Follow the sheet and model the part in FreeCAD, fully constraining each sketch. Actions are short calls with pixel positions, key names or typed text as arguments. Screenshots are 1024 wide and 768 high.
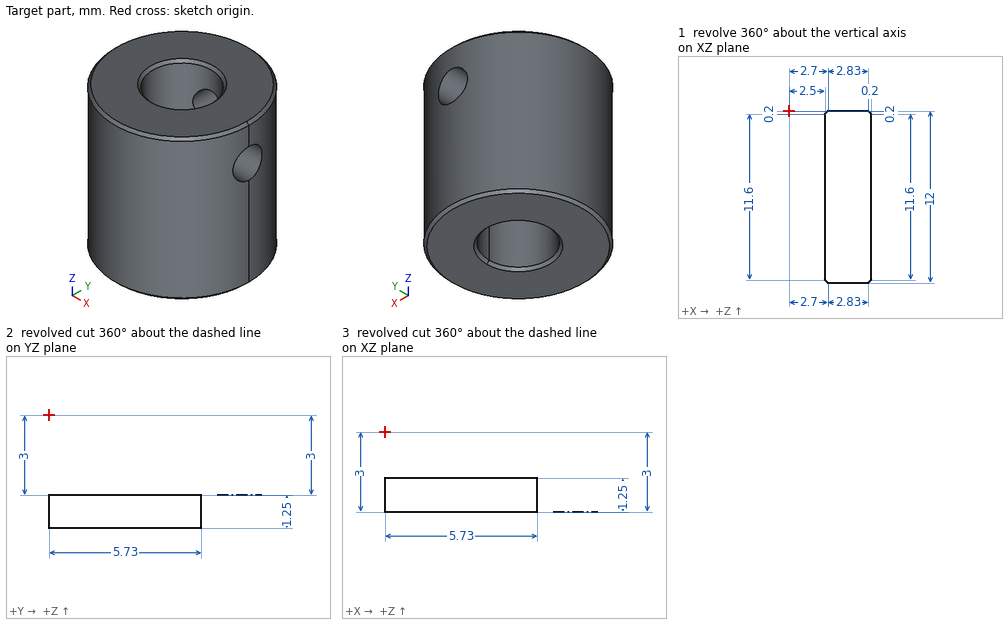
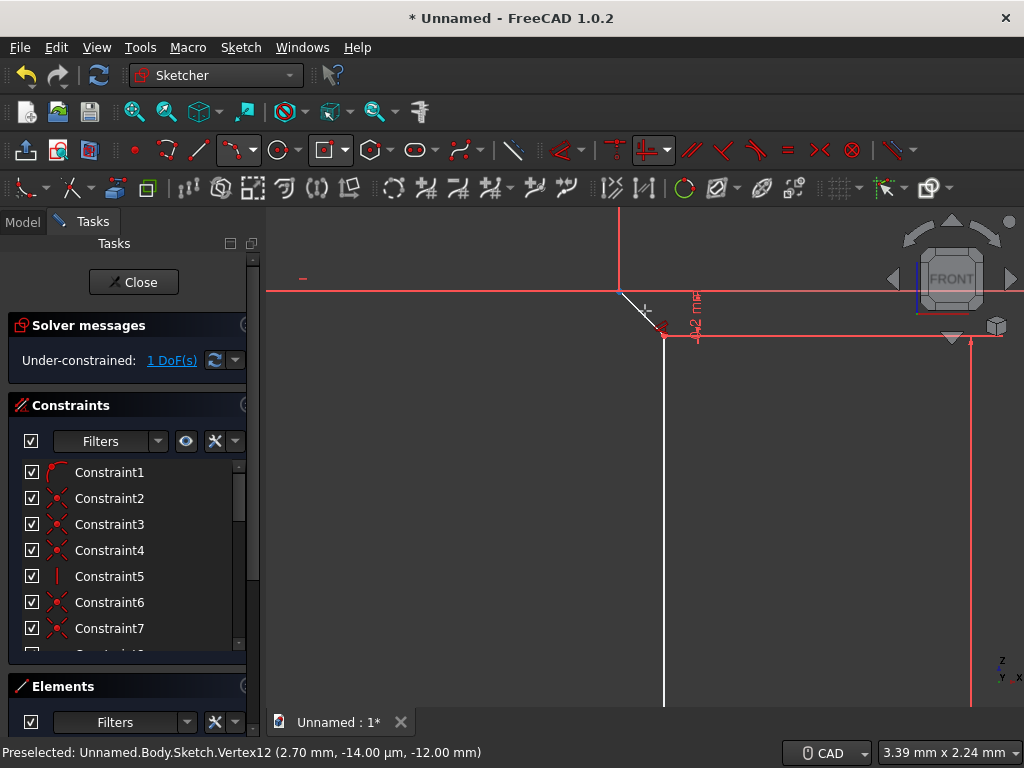
click(637, 309)
click(642, 257)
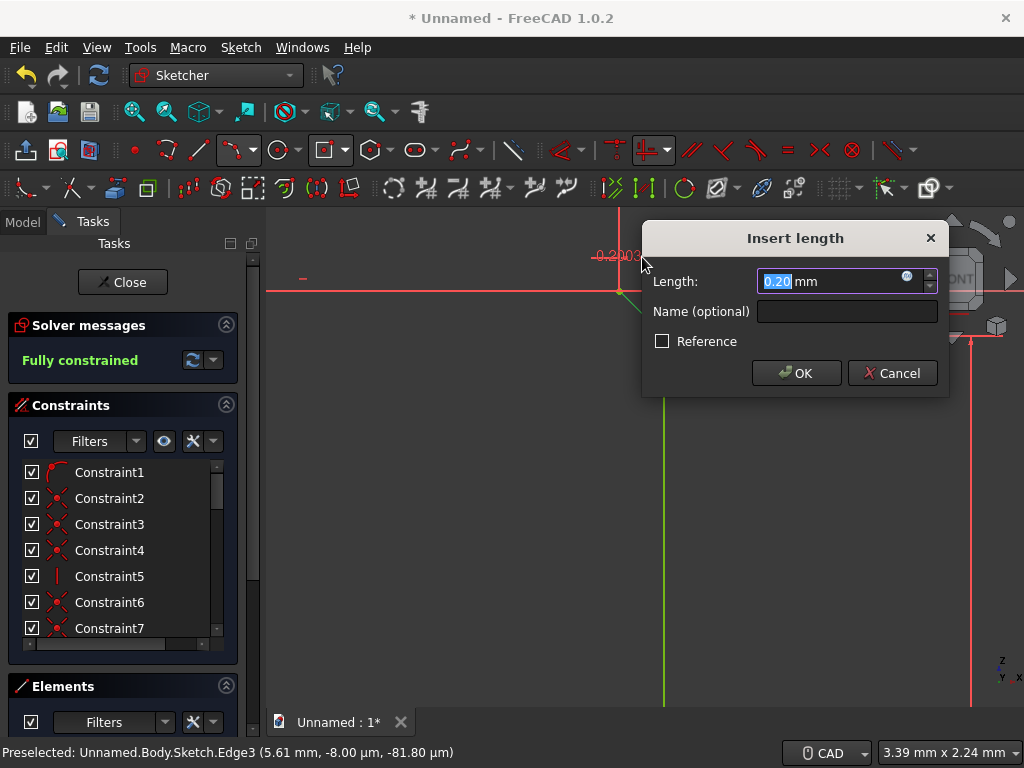
text(0.2)
key(Return)
key(Escape)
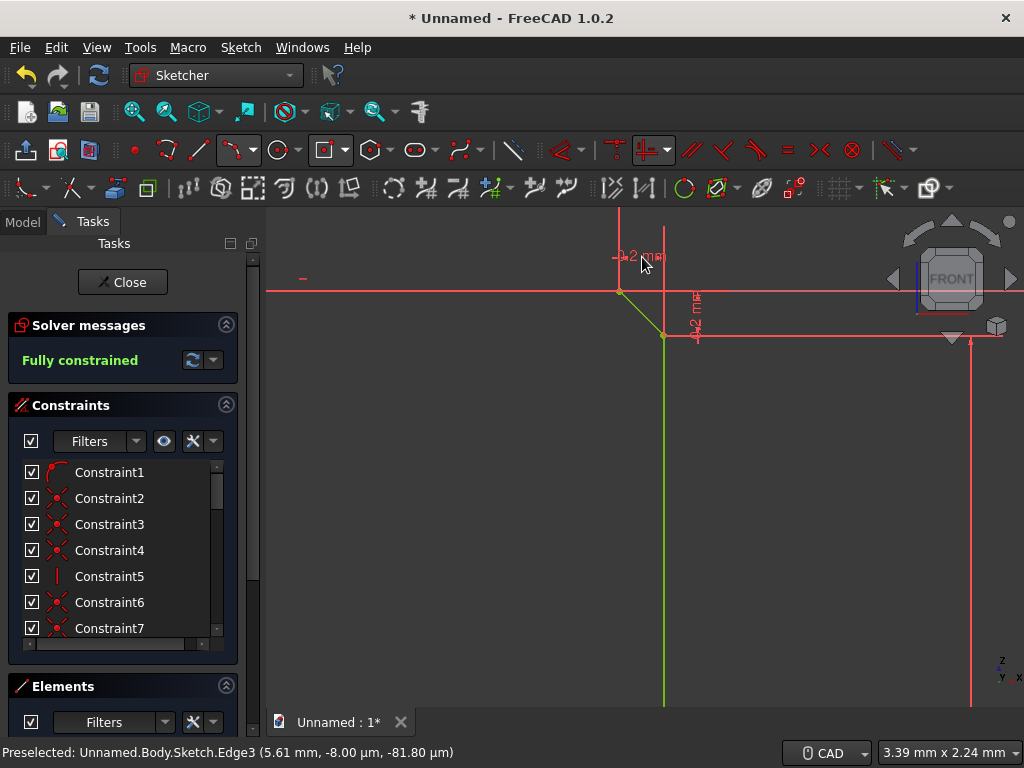
click(123, 282)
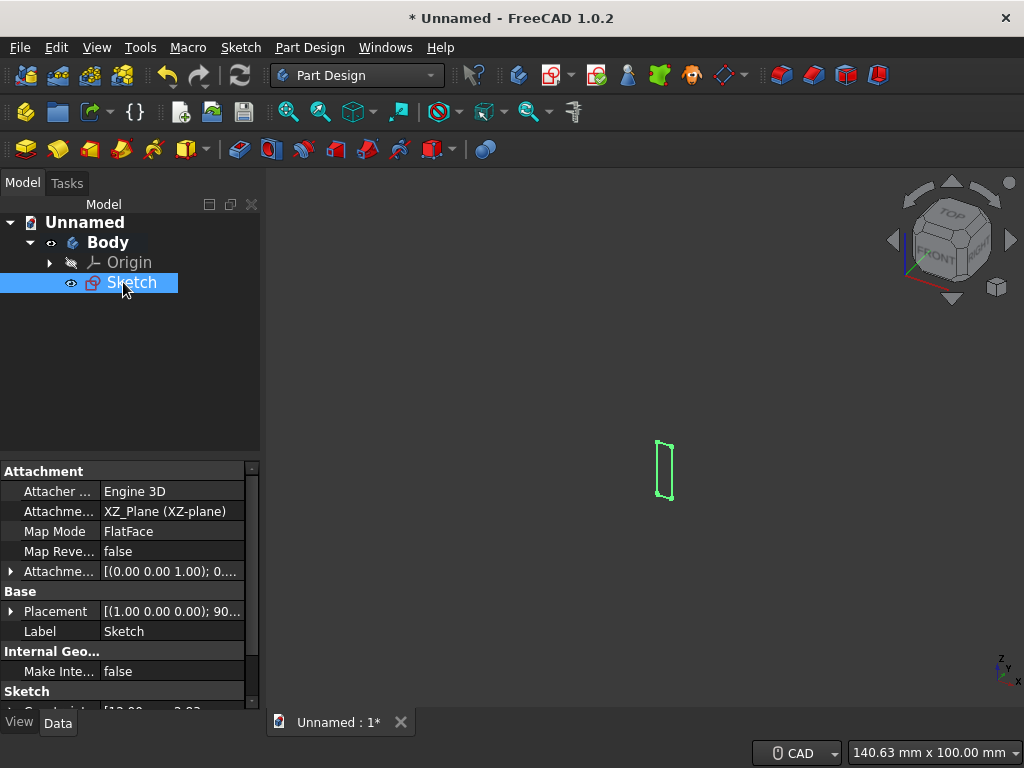
click(58, 150)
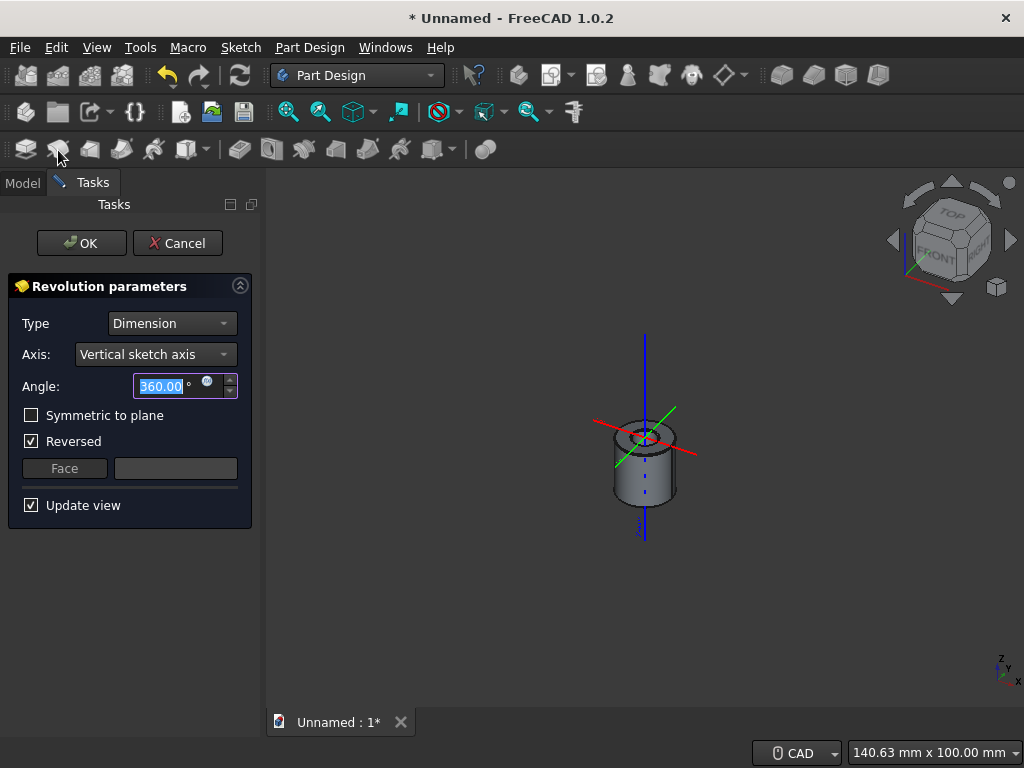
click(82, 243)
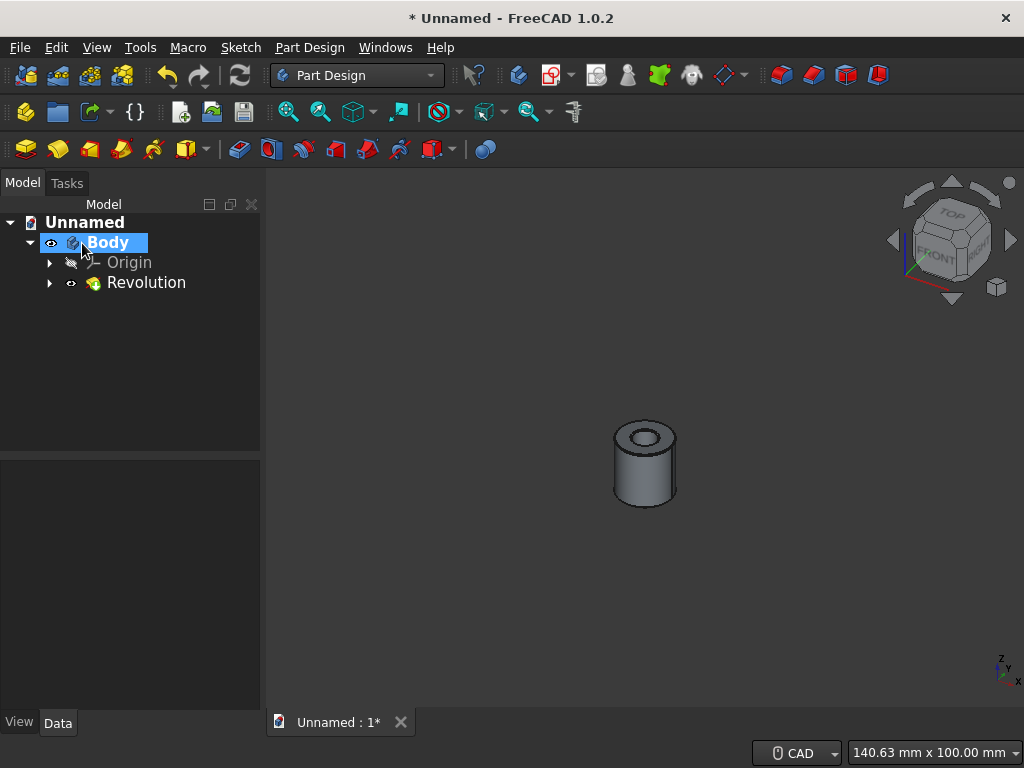
click(290, 112)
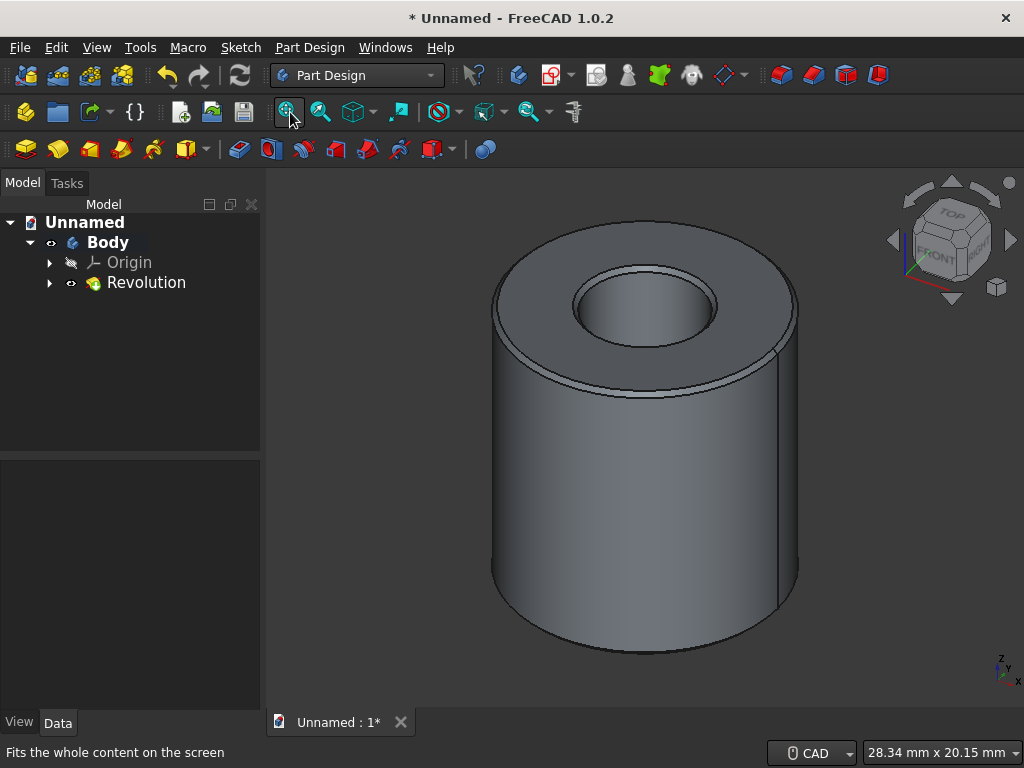
click(552, 76)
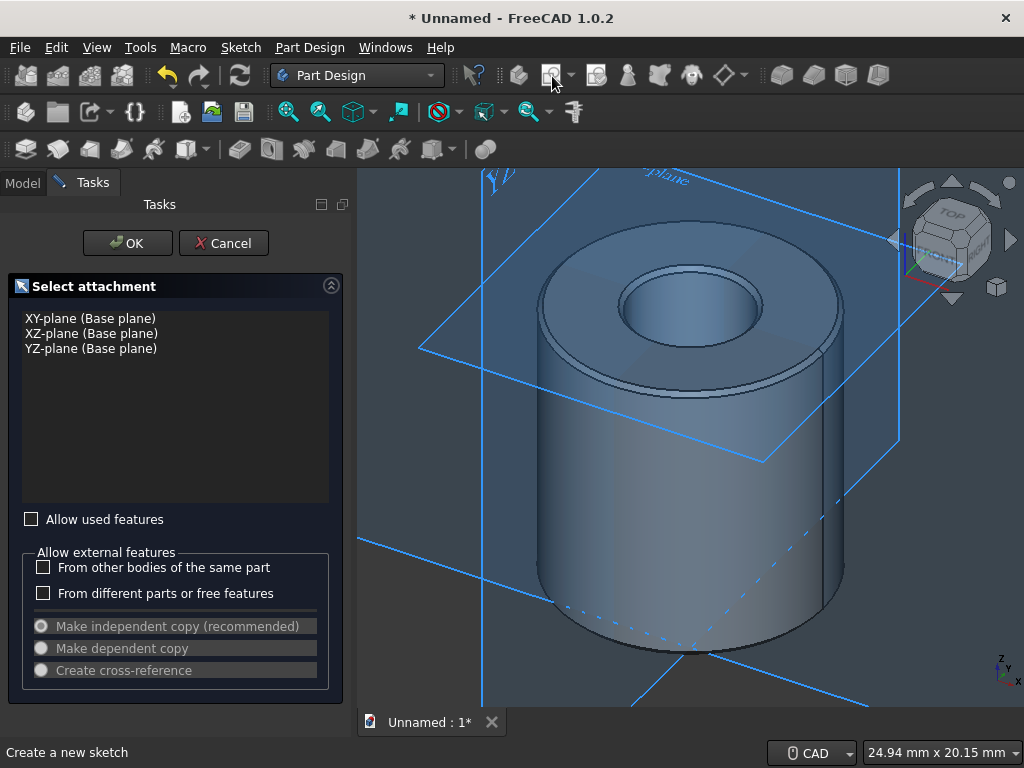
click(82, 348)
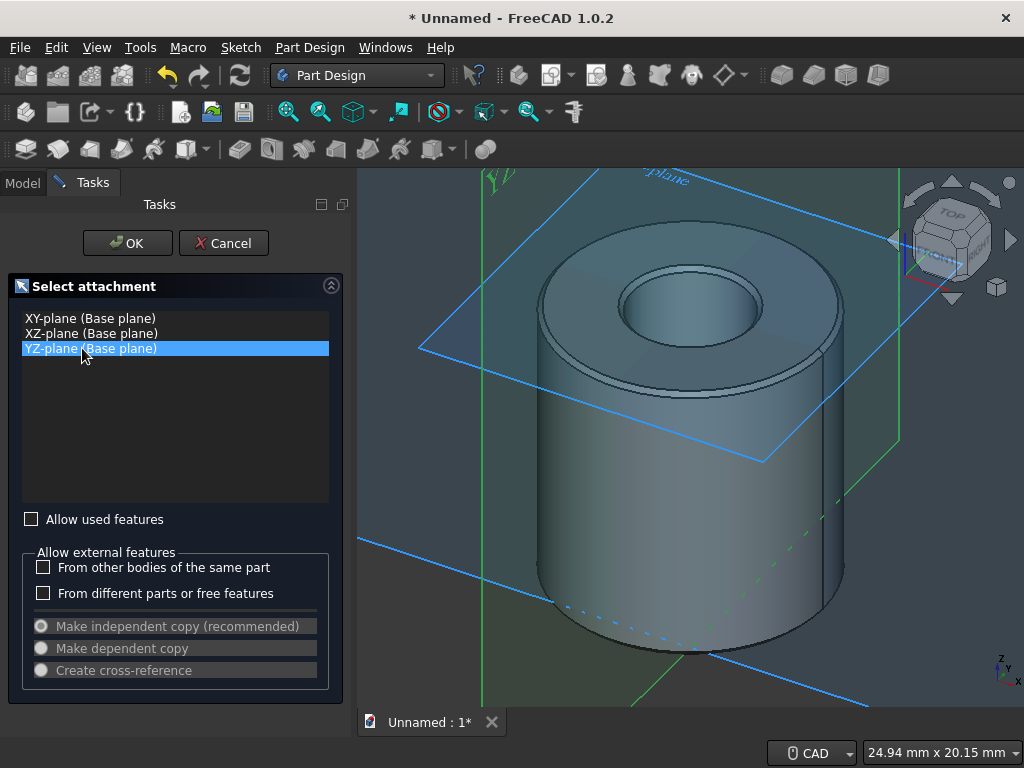
click(128, 243)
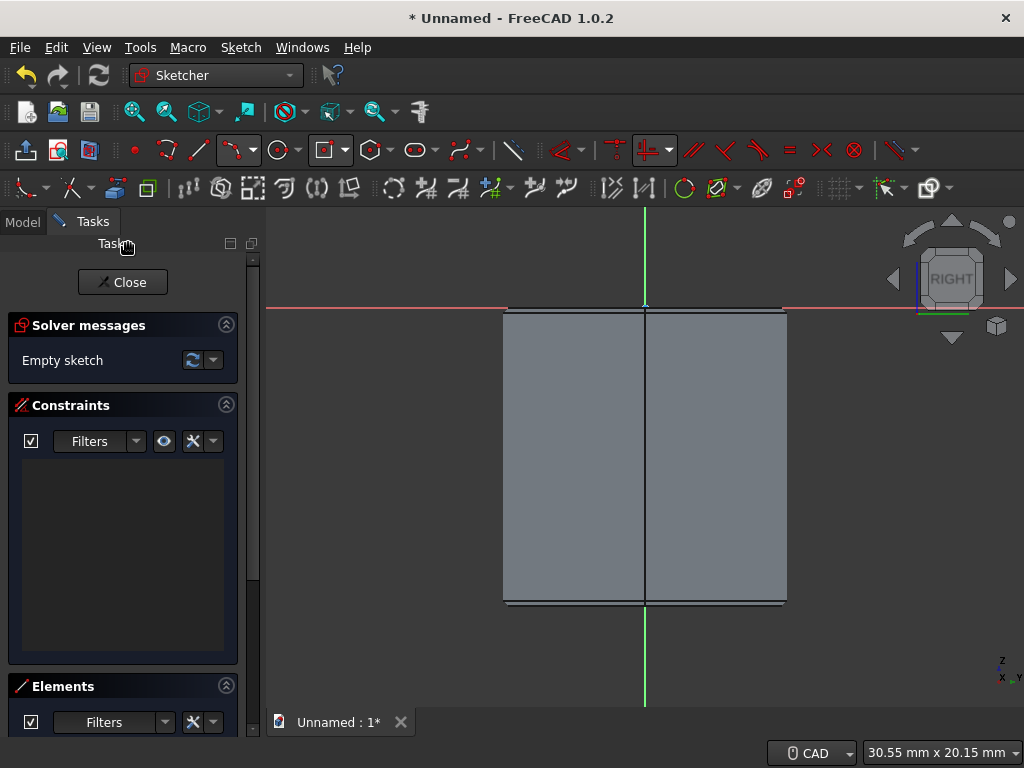
click(90, 150)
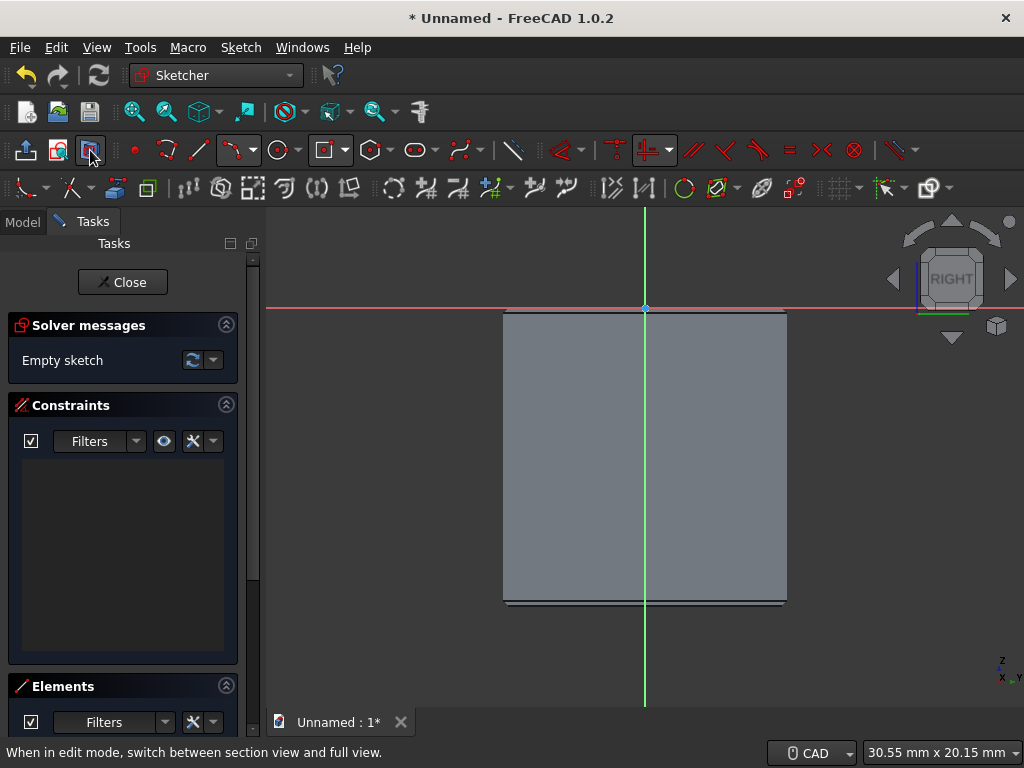
scroll(859, 244, up, 3)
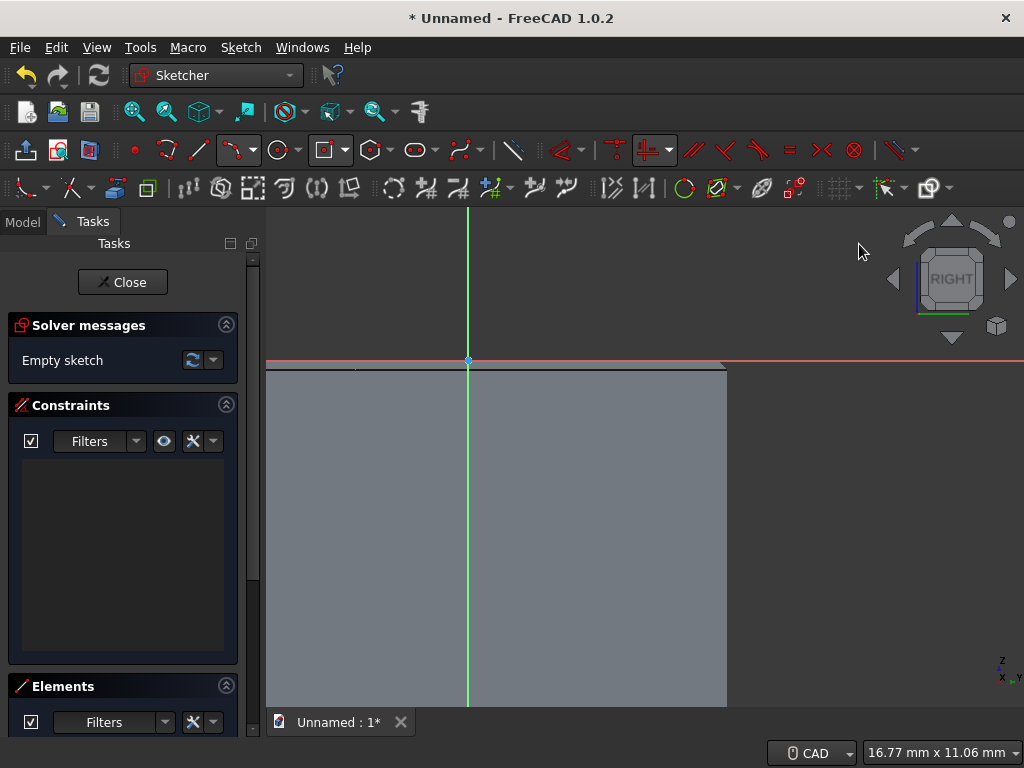
key(g)
key(r)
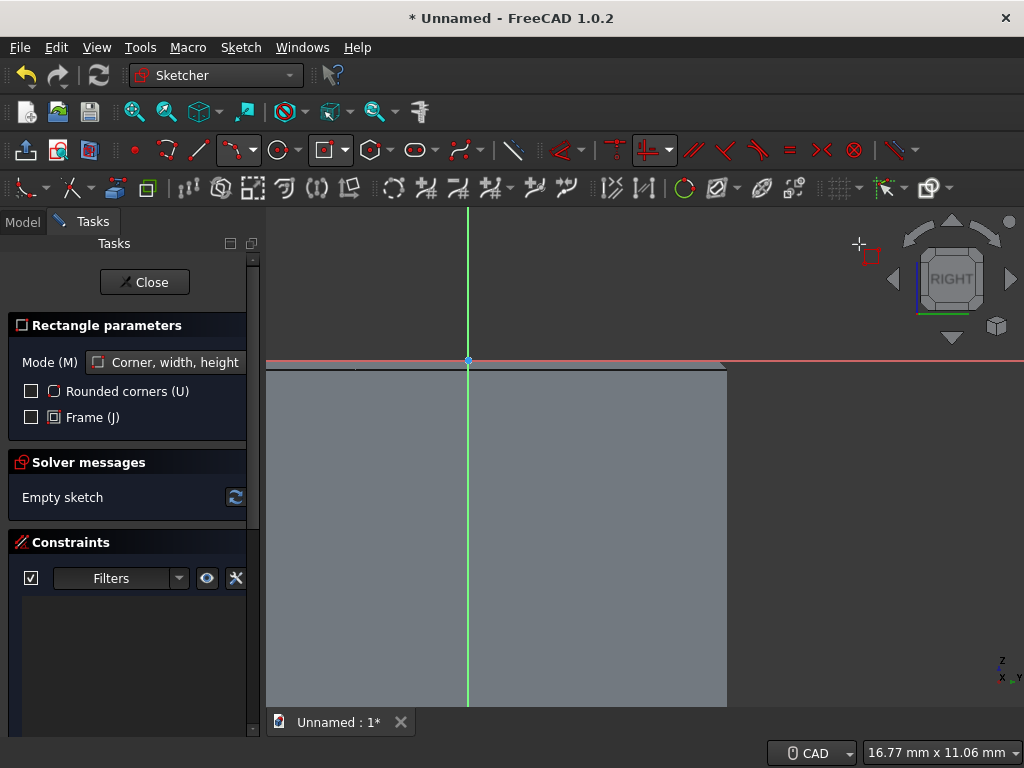
click(468, 496)
move(727, 553)